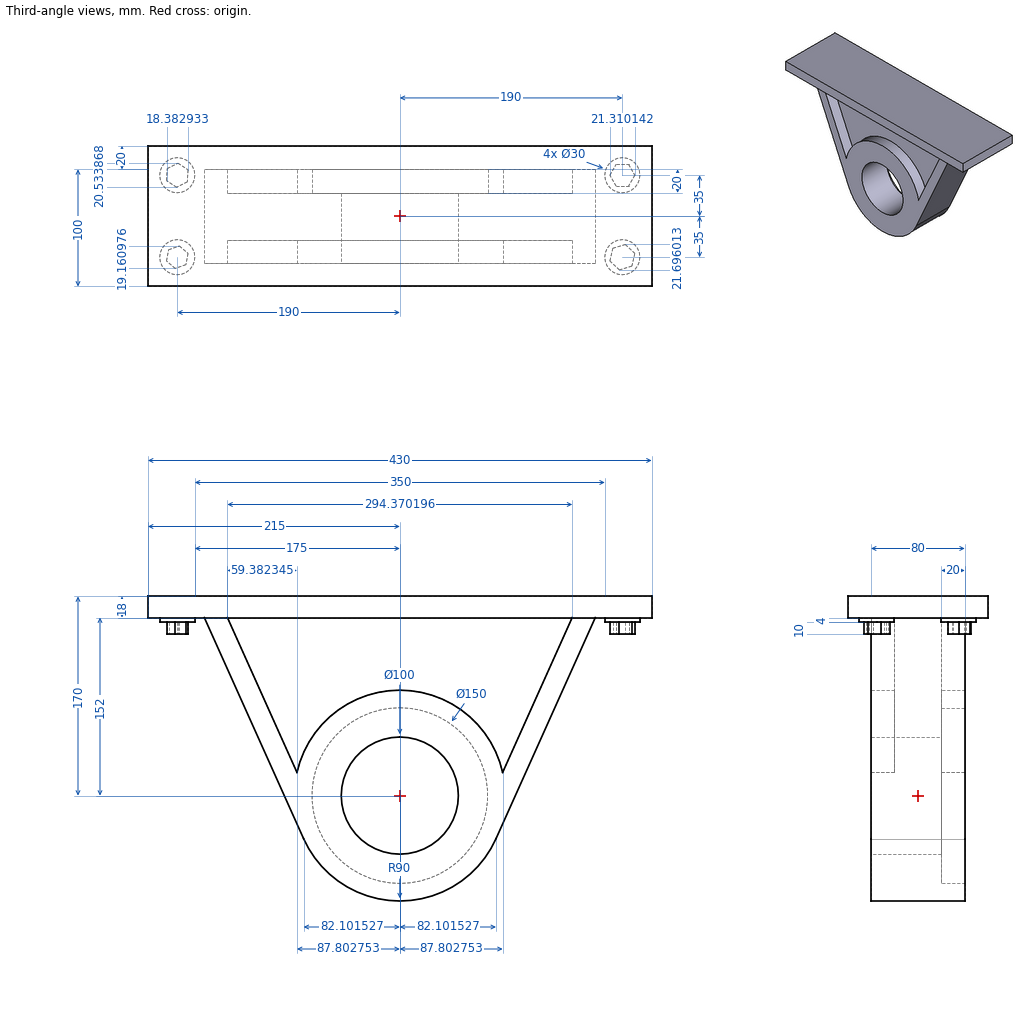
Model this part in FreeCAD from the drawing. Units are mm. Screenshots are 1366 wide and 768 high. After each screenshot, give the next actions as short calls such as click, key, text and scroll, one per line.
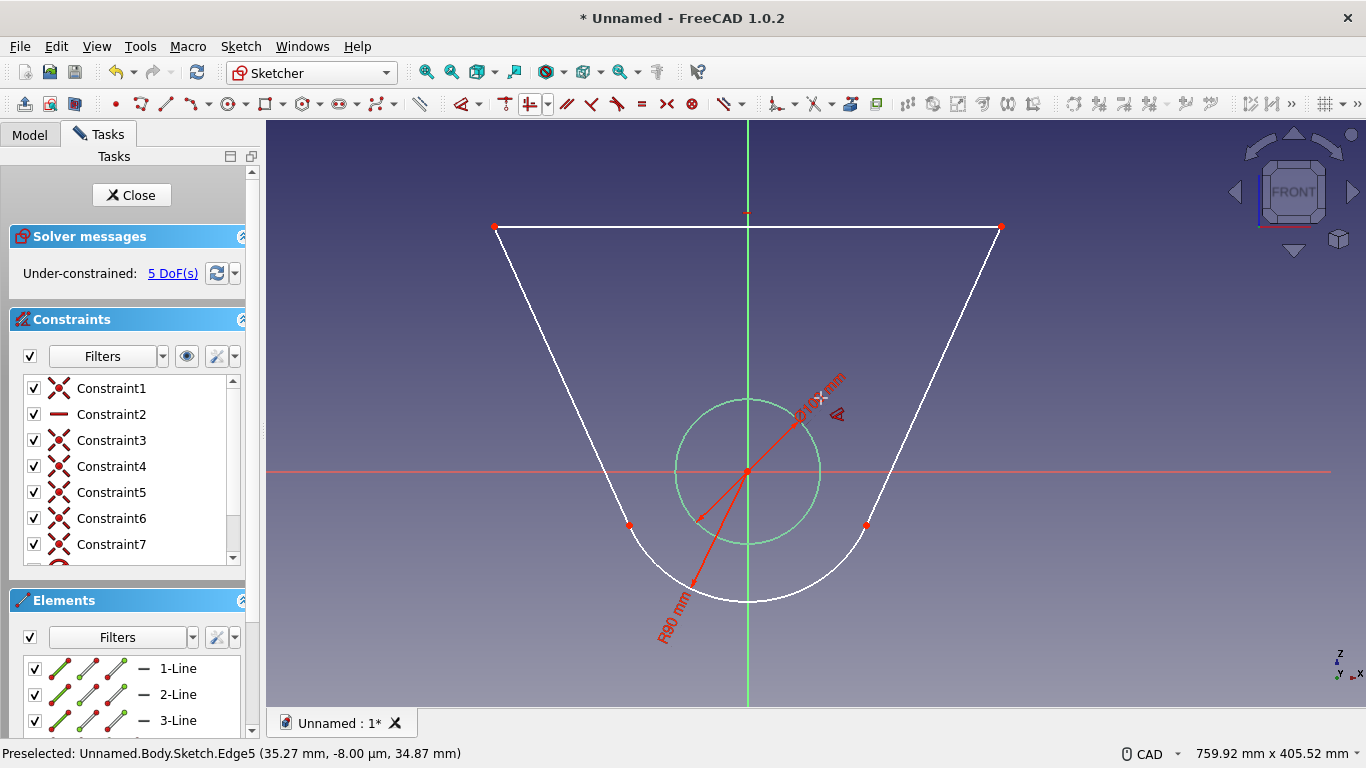
click(646, 227)
click(631, 193)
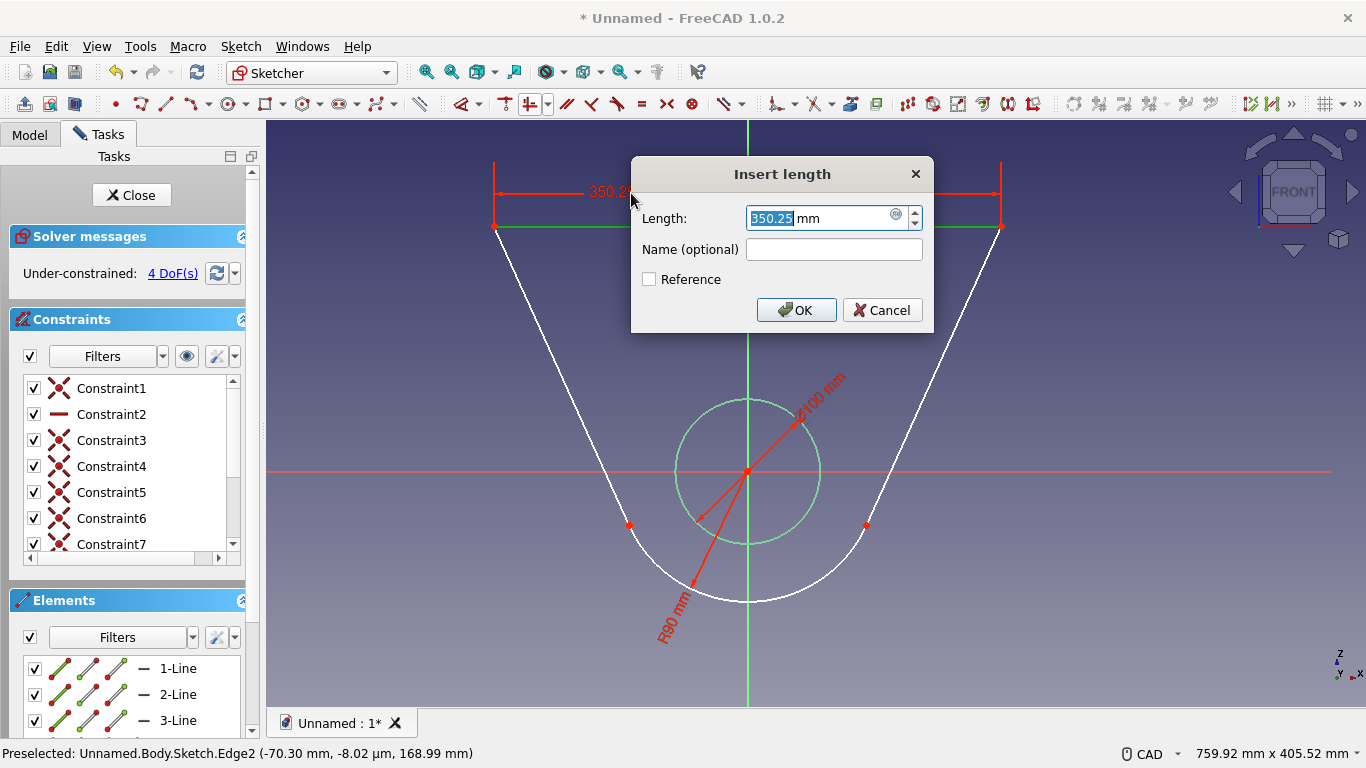
text(350)
key(Return)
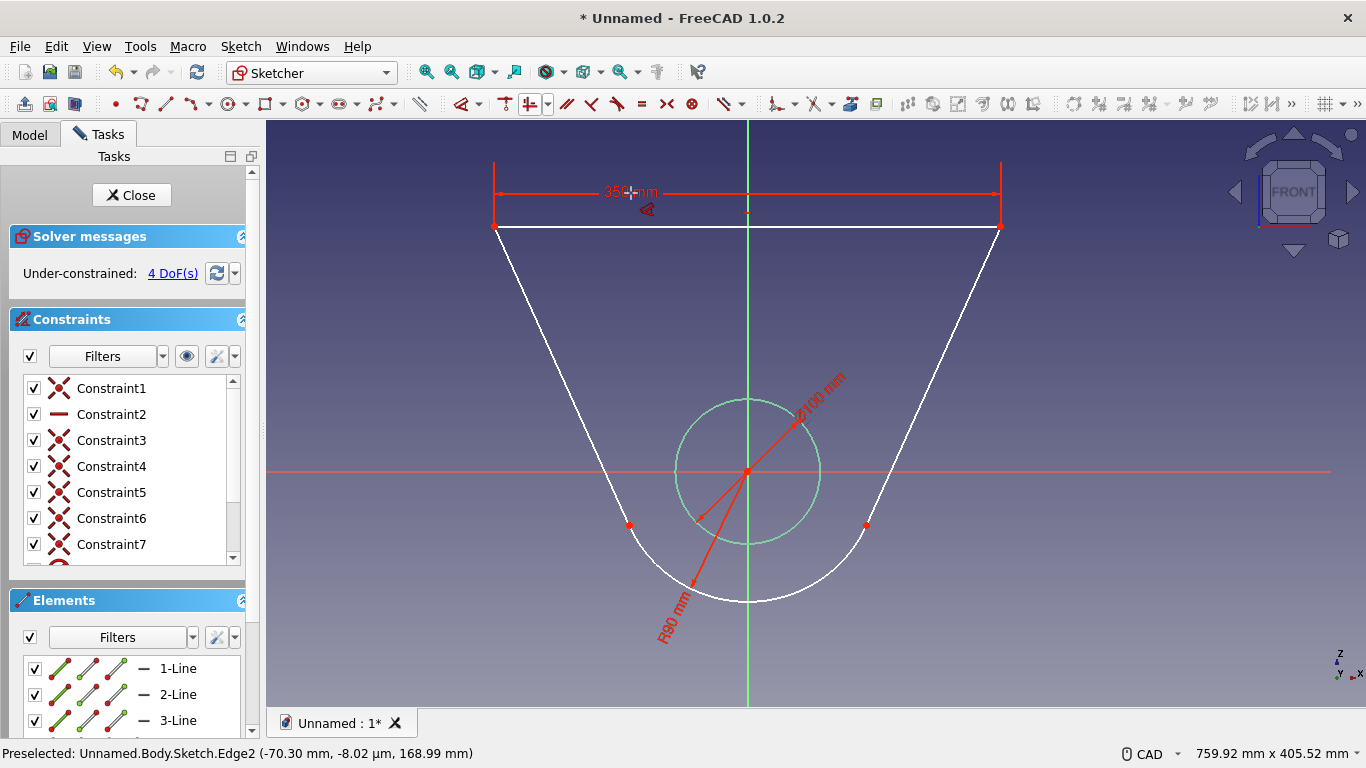
click(494, 227)
click(532, 193)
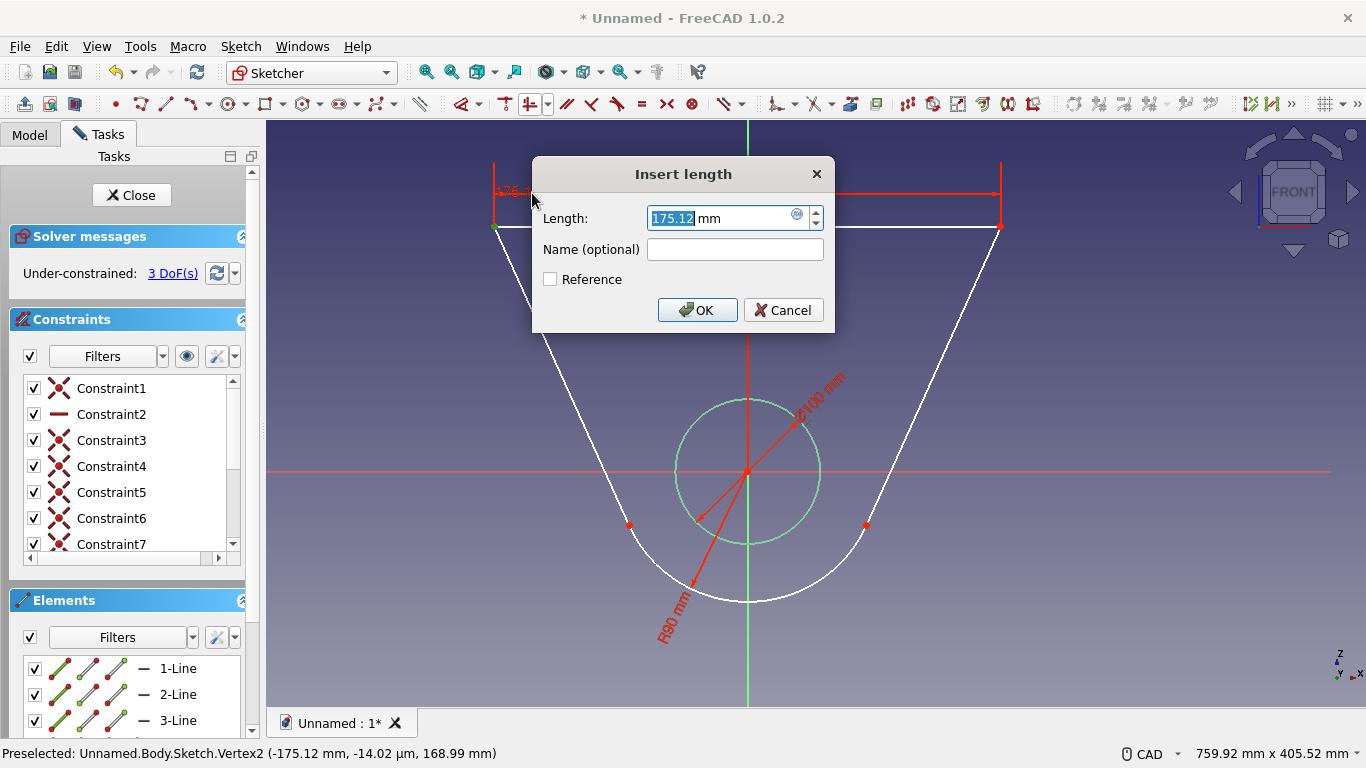
text(175)
key(Return)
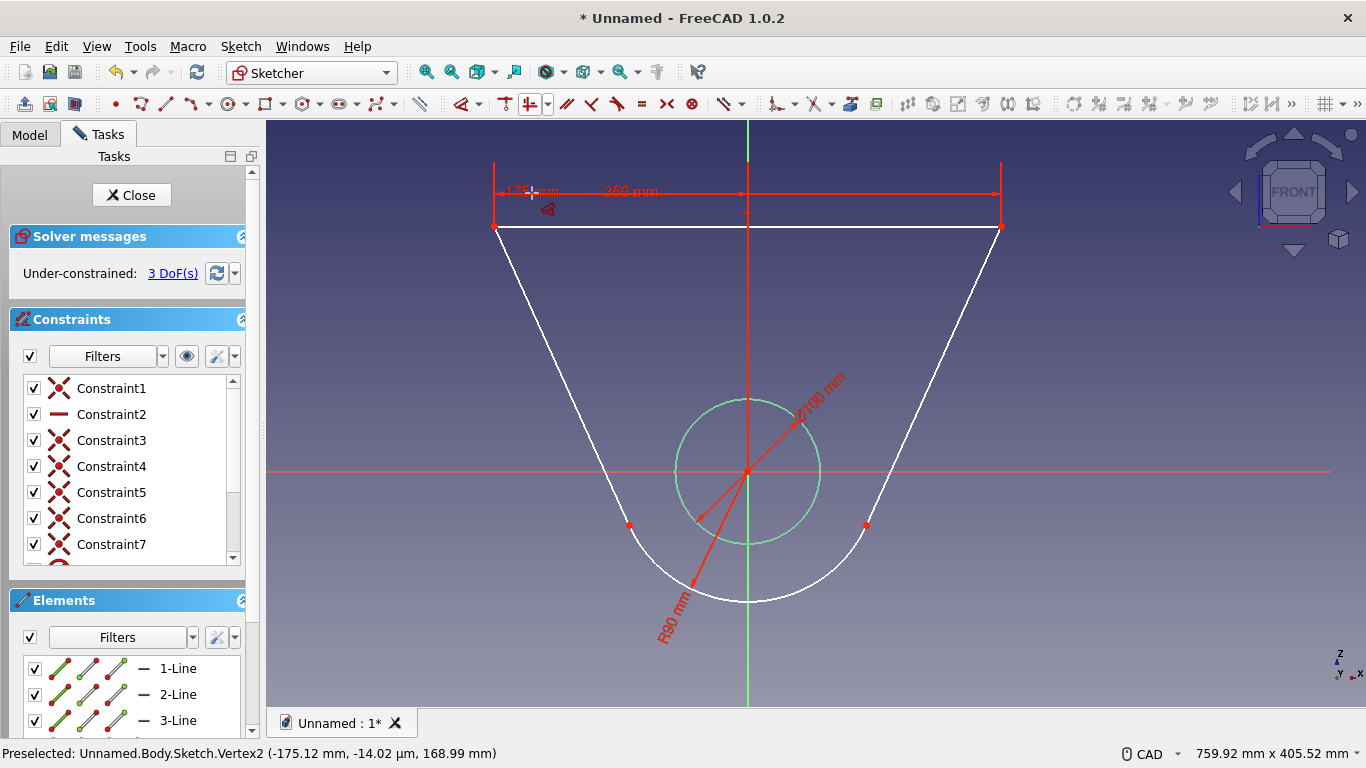
click(494, 227)
click(460, 349)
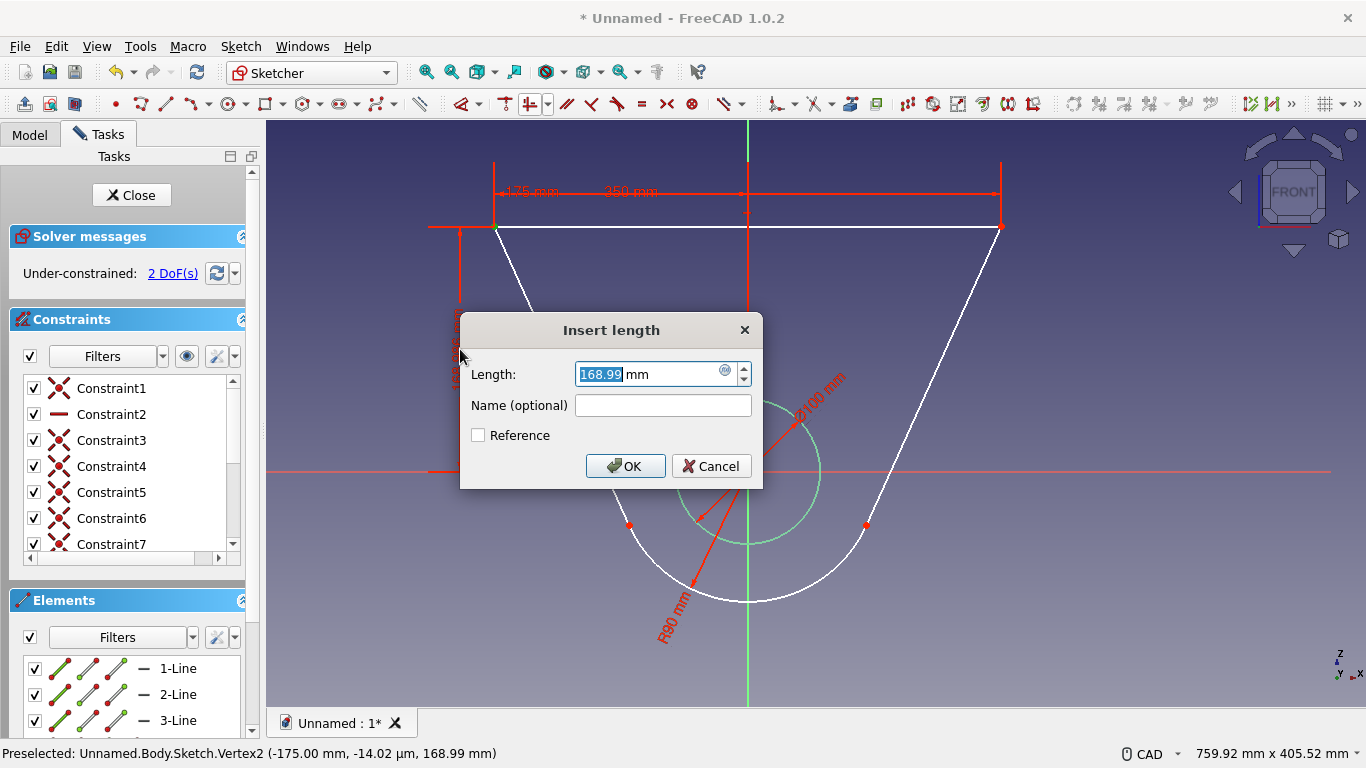
text(170)
key(Return)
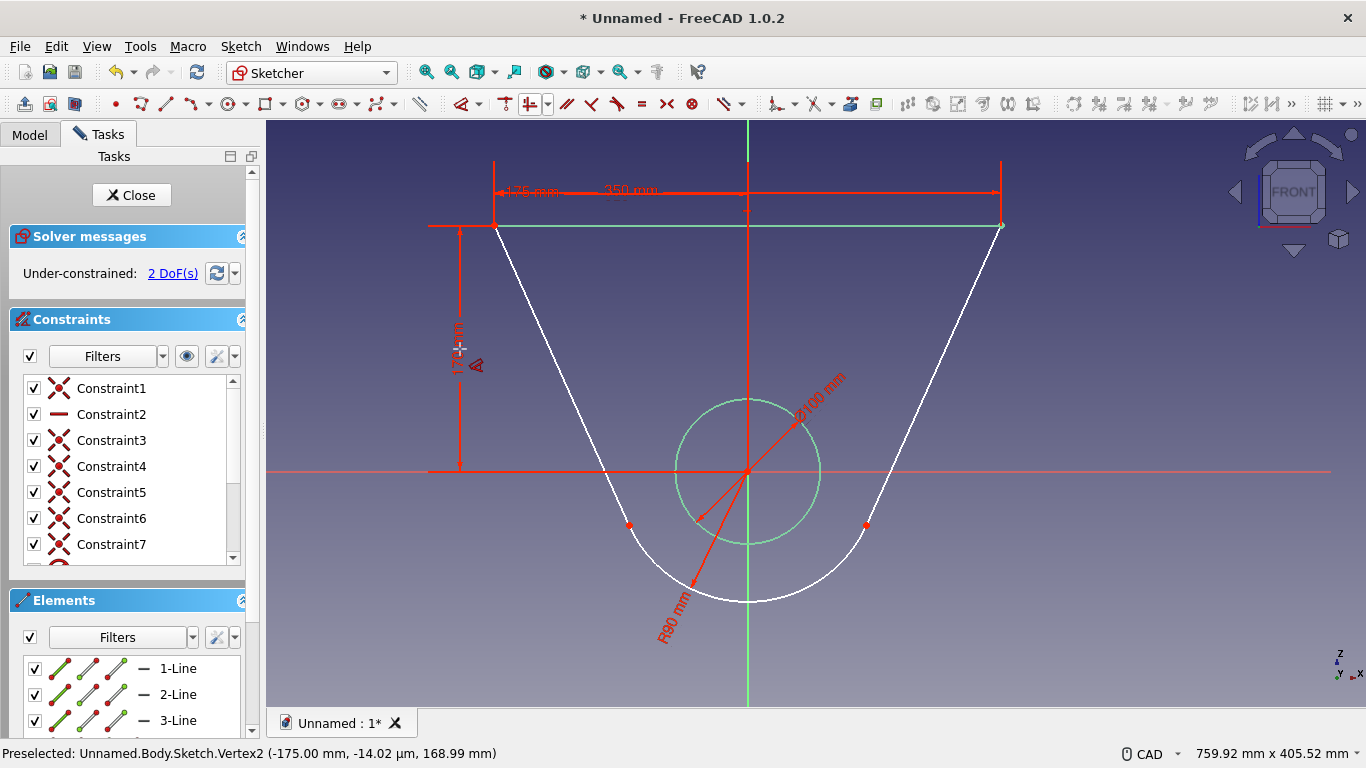
click(629, 526)
click(689, 560)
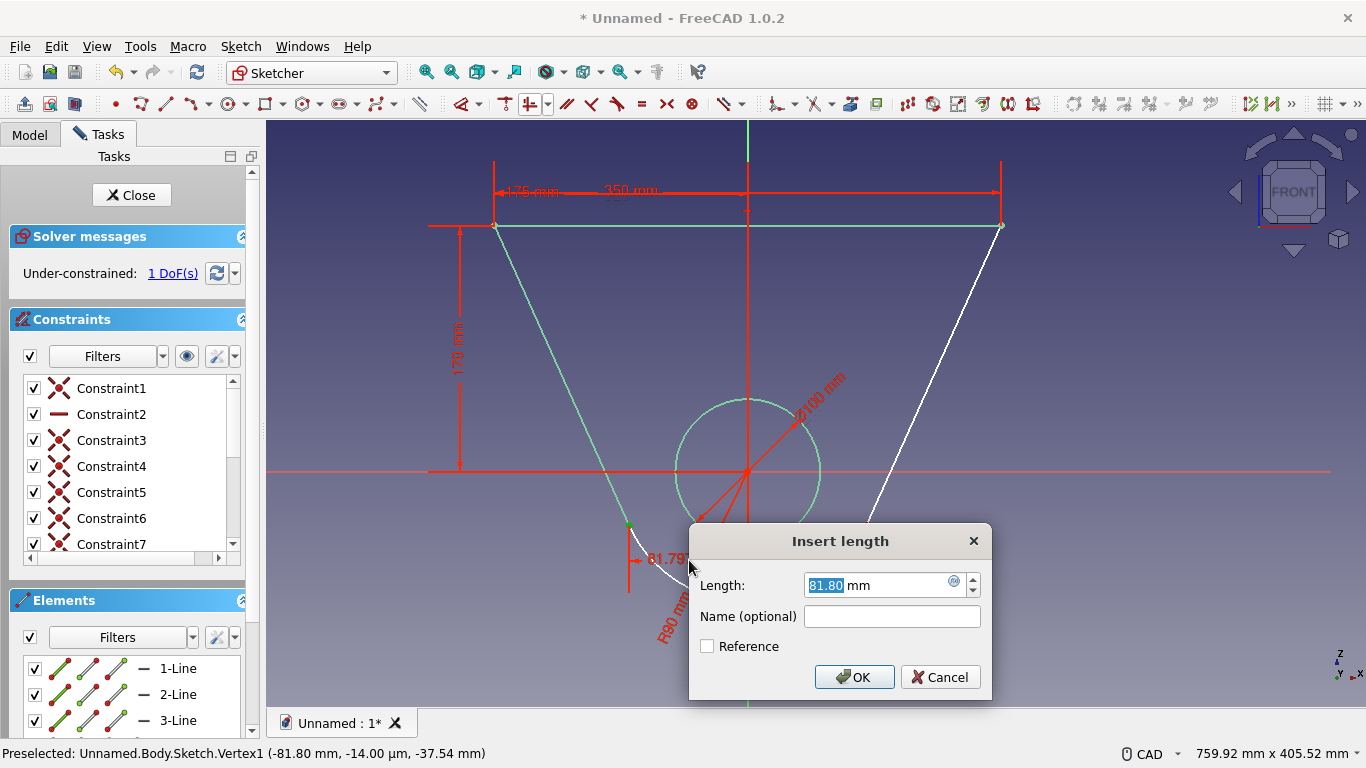
text(82.101527)
key(Return)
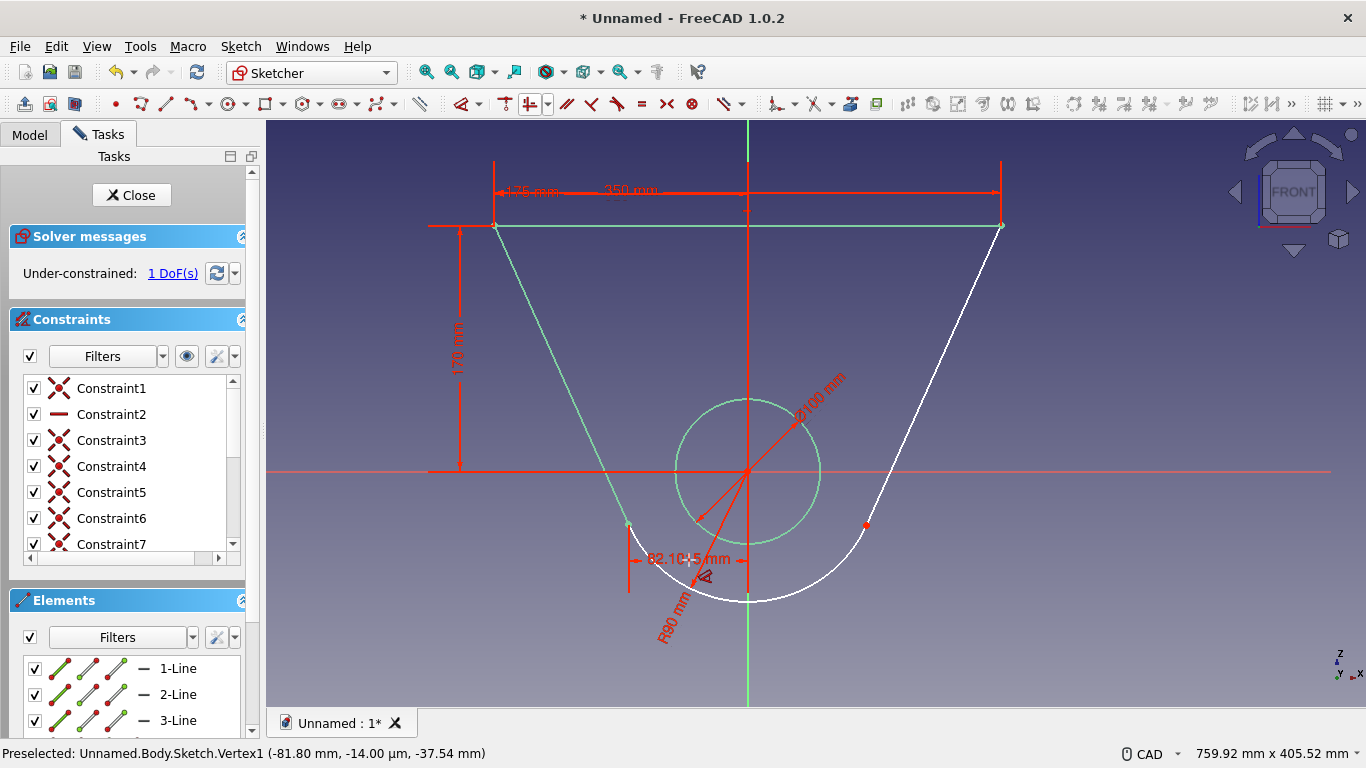
click(866, 526)
click(807, 560)